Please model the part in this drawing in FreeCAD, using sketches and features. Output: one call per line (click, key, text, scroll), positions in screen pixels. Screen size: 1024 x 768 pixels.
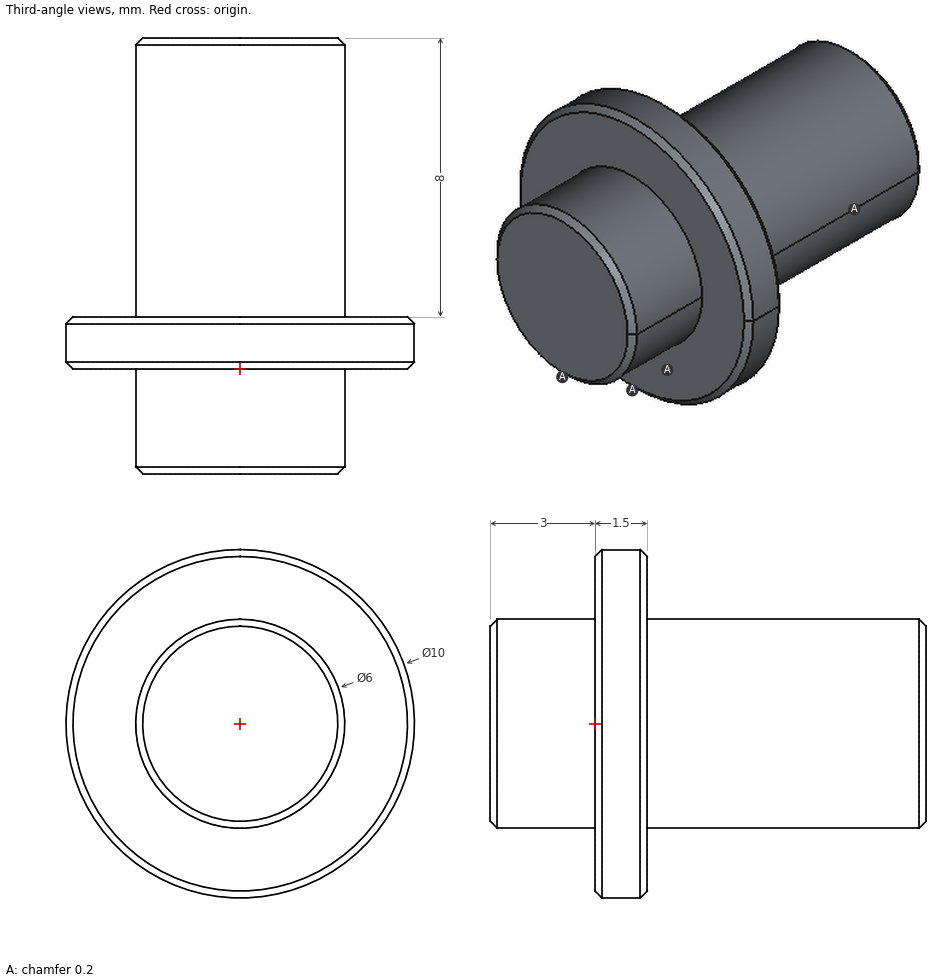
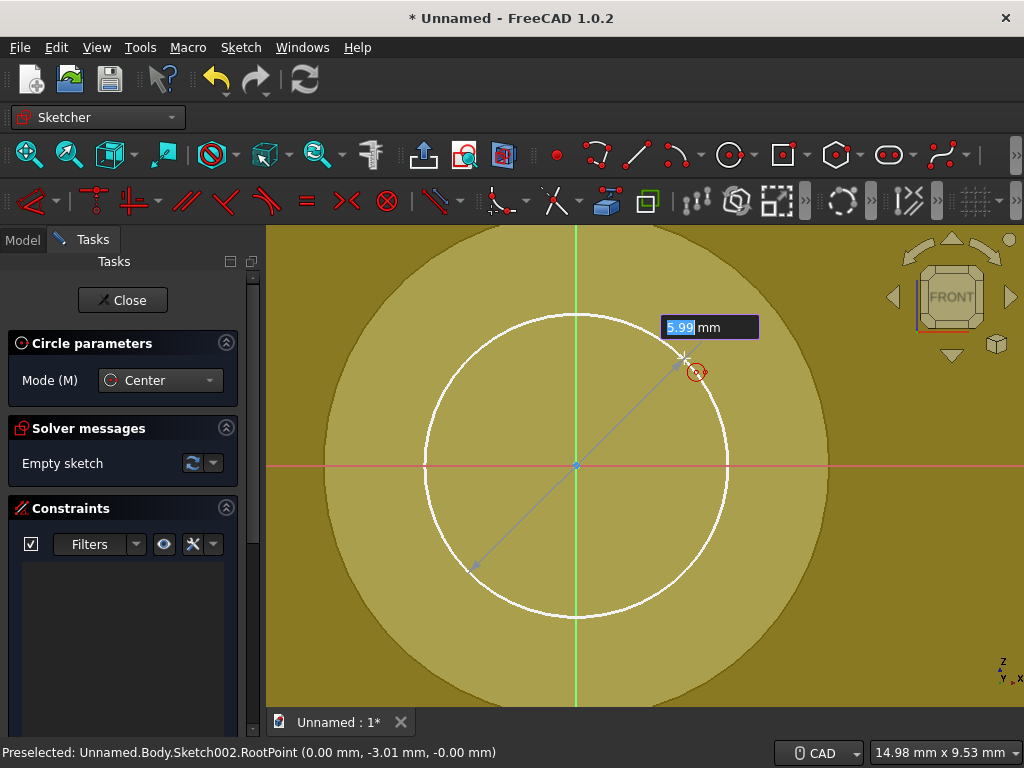
text(6)
key(Return)
key(Escape)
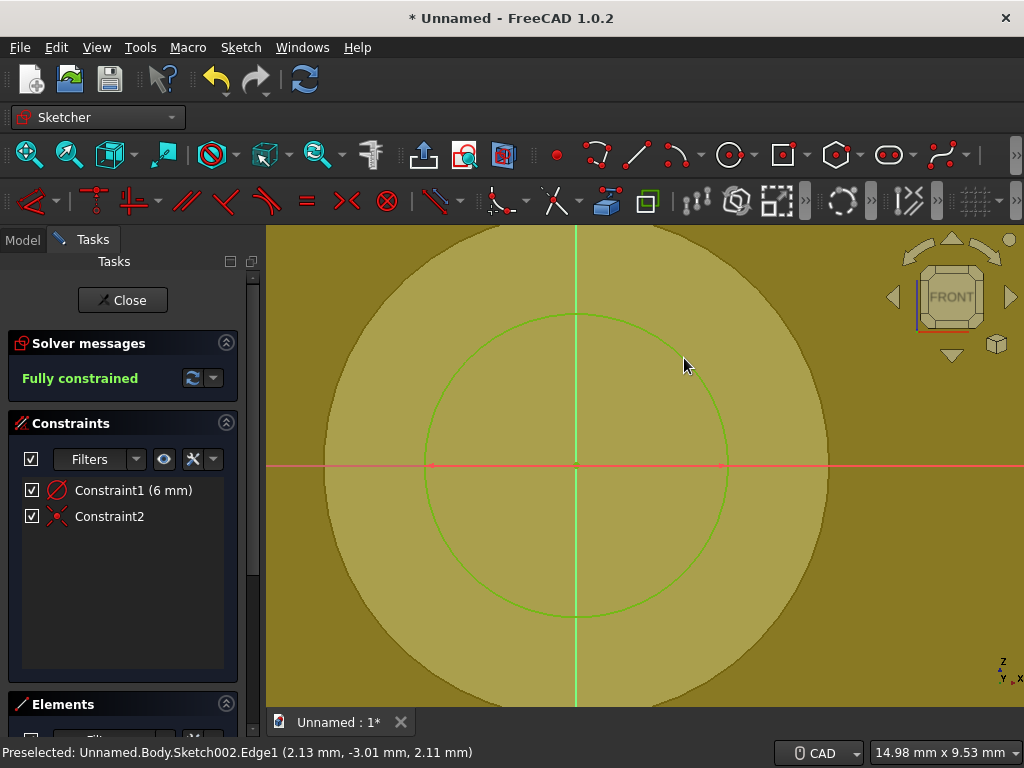
click(123, 300)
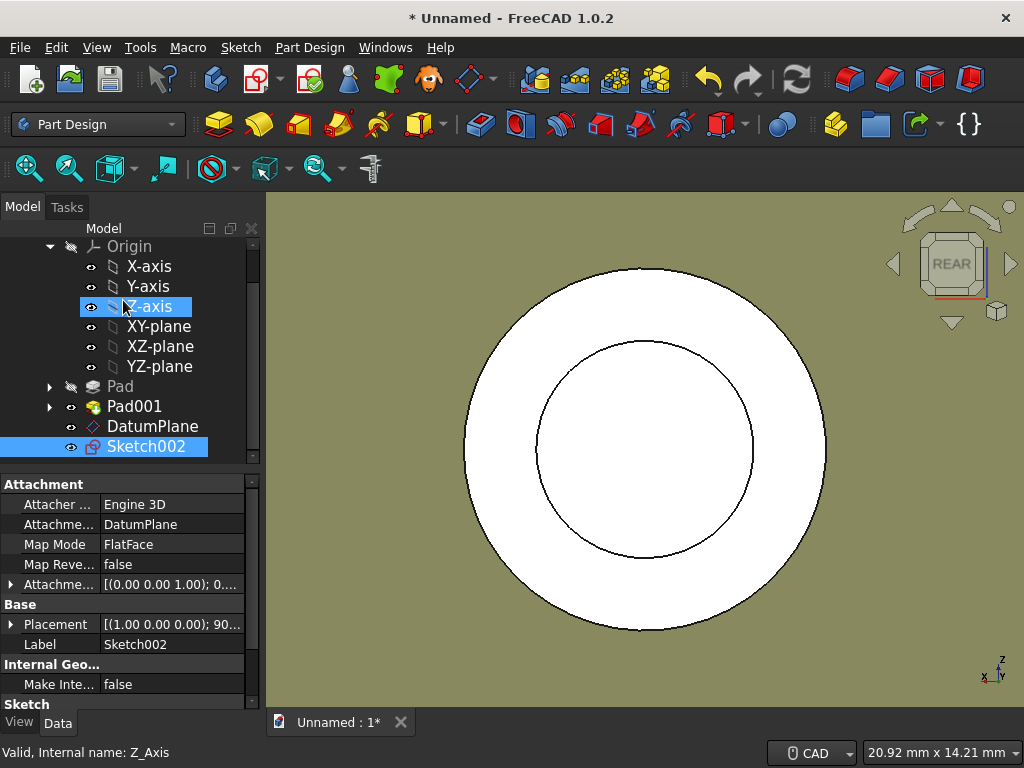
click(220, 124)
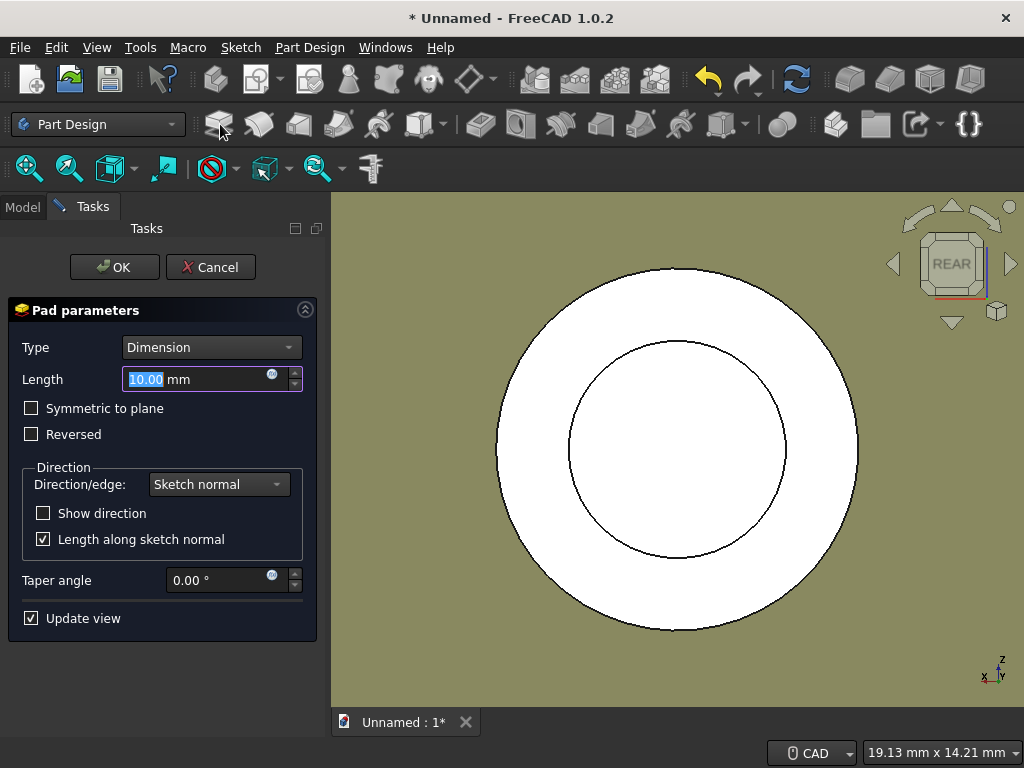
text(3)
key(Tab)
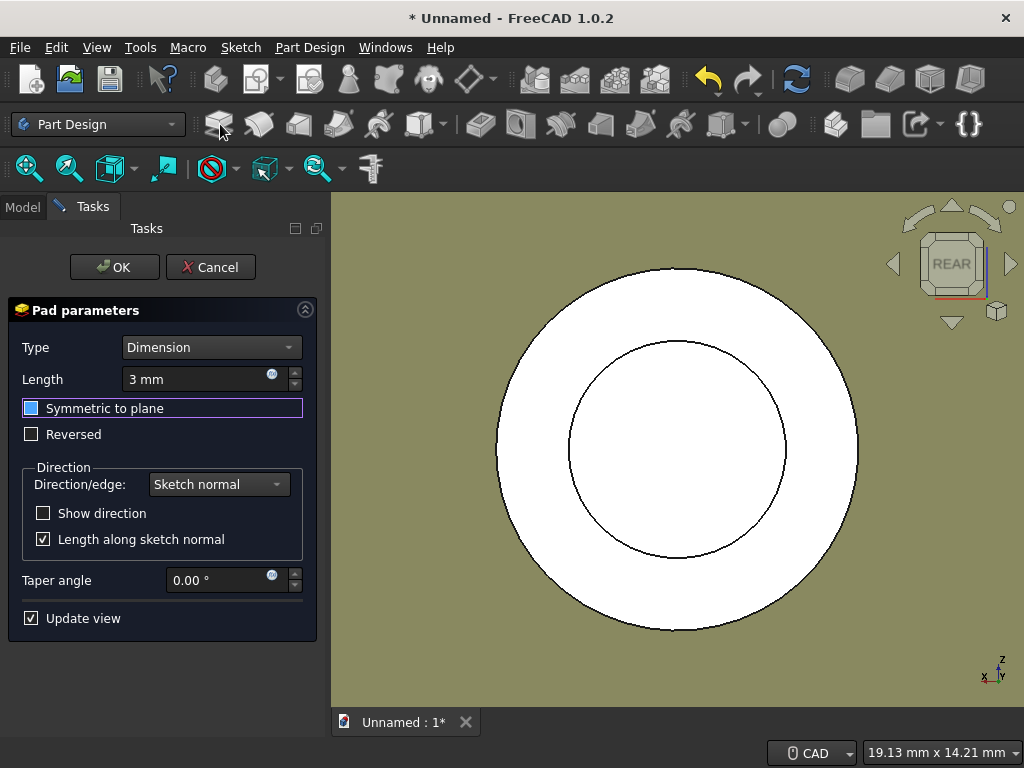
click(30, 434)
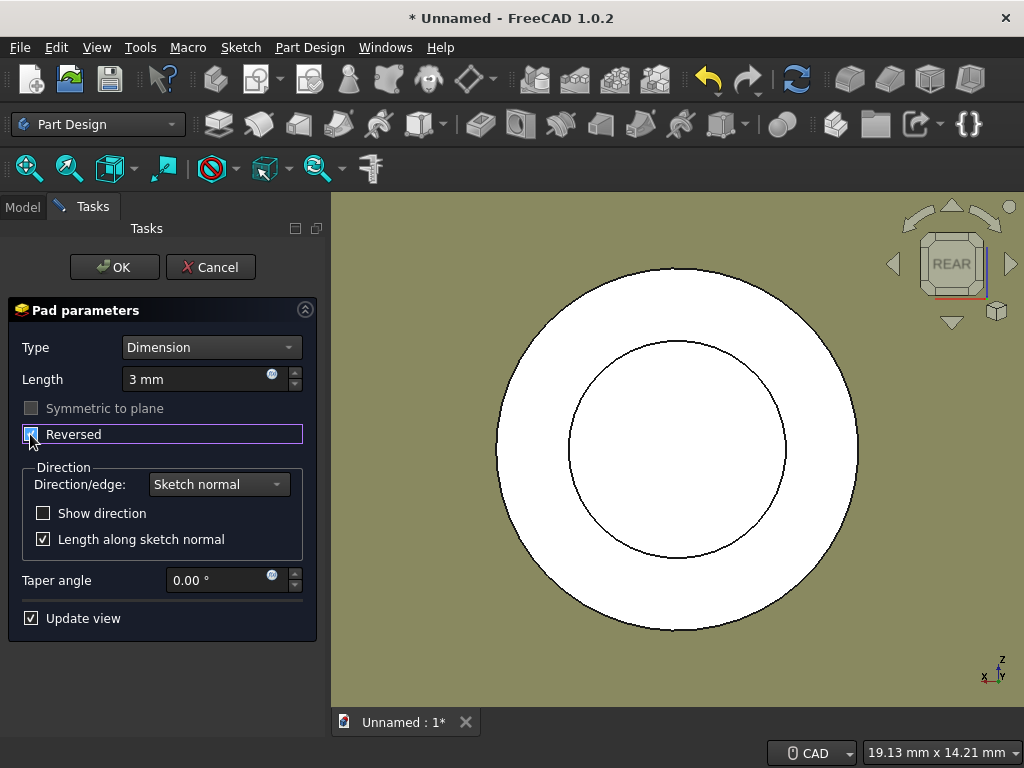
click(115, 267)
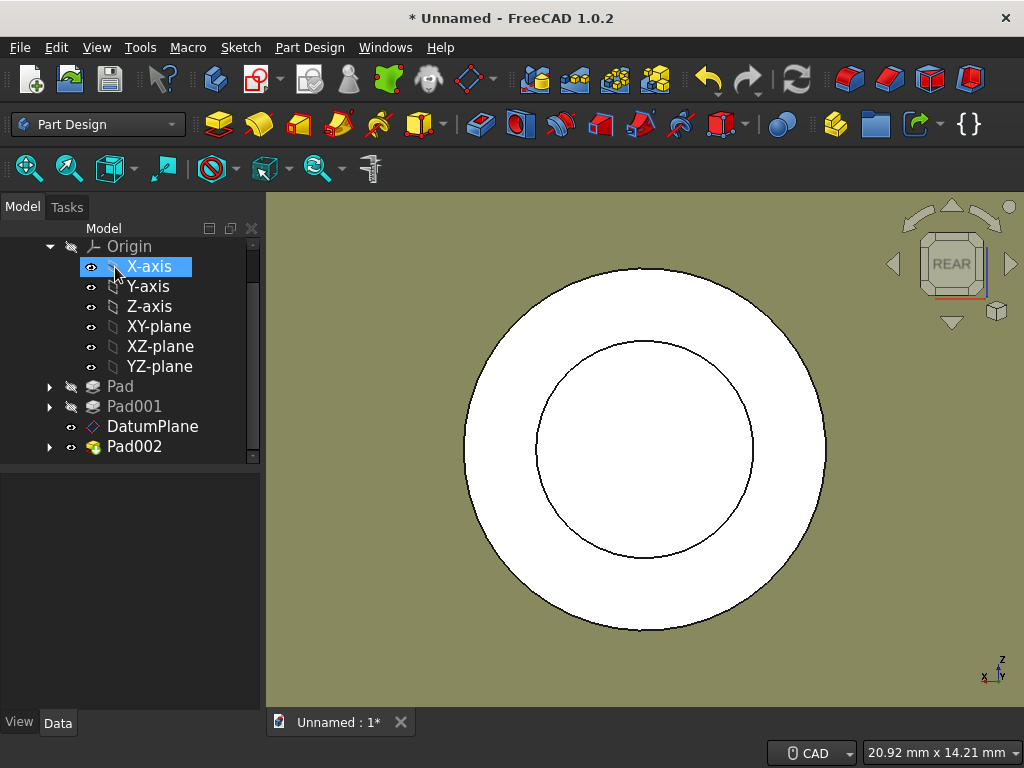
click(116, 427)
key(space)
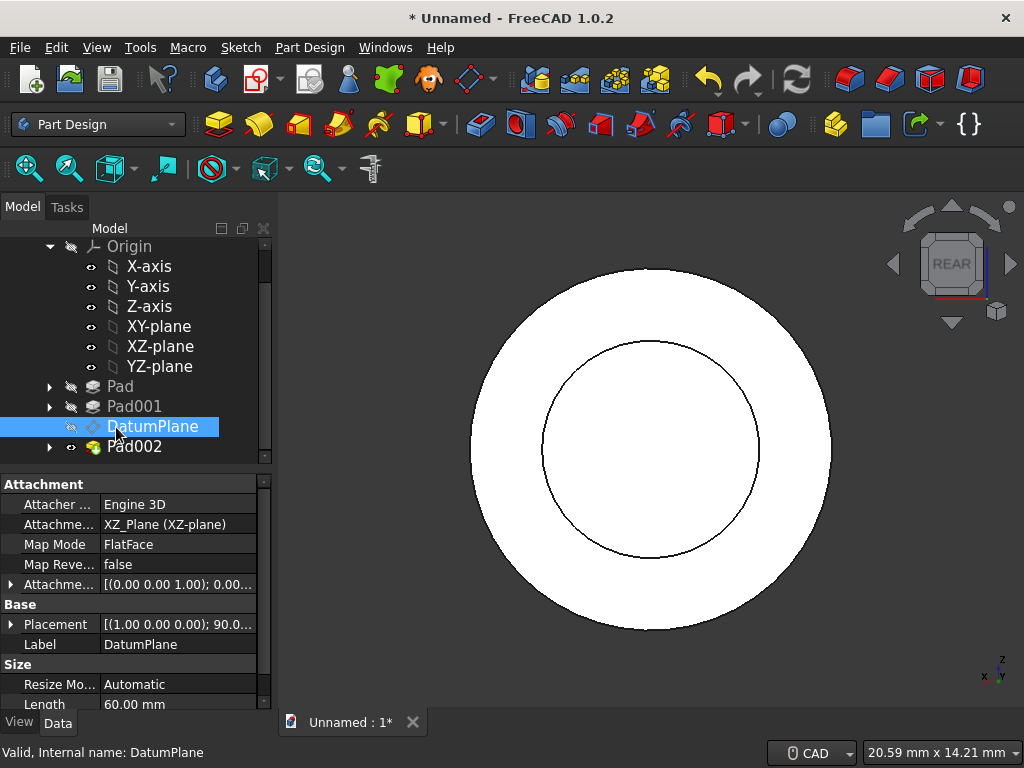
click(832, 448)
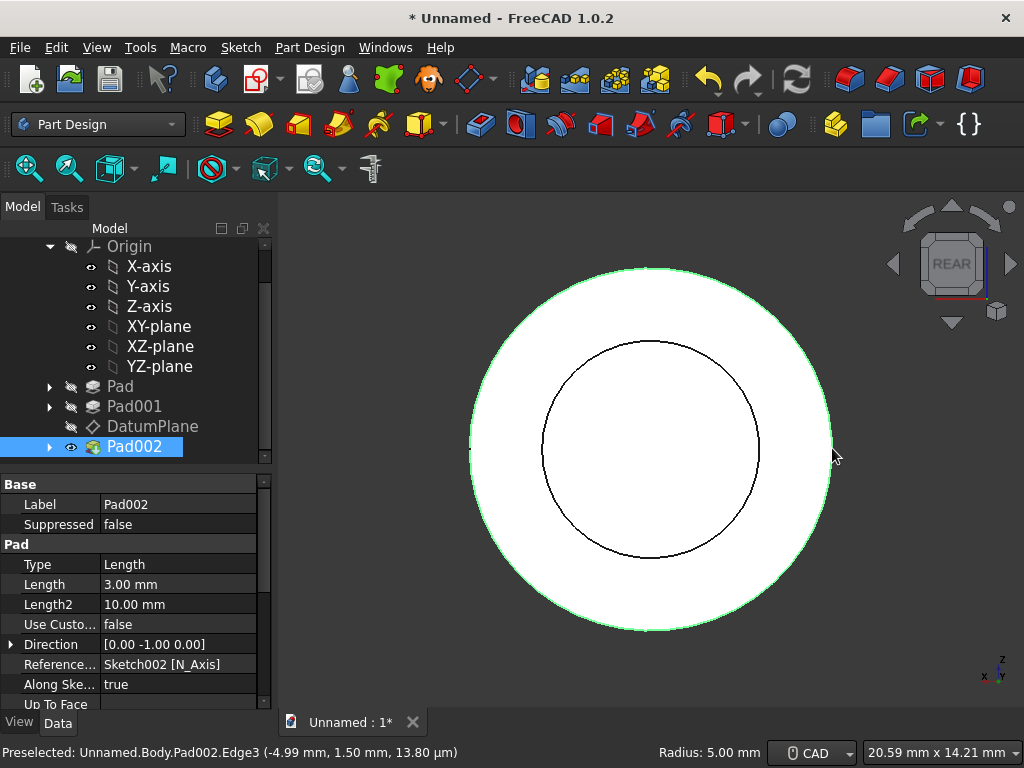
click(759, 448, ctrl)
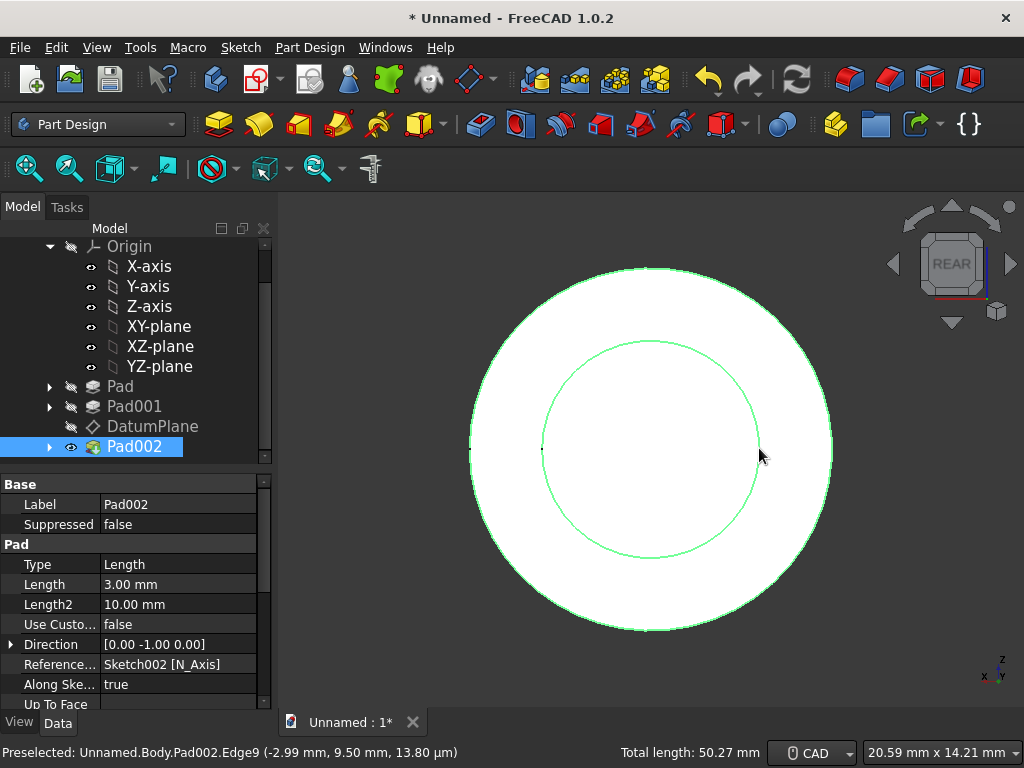
key(0)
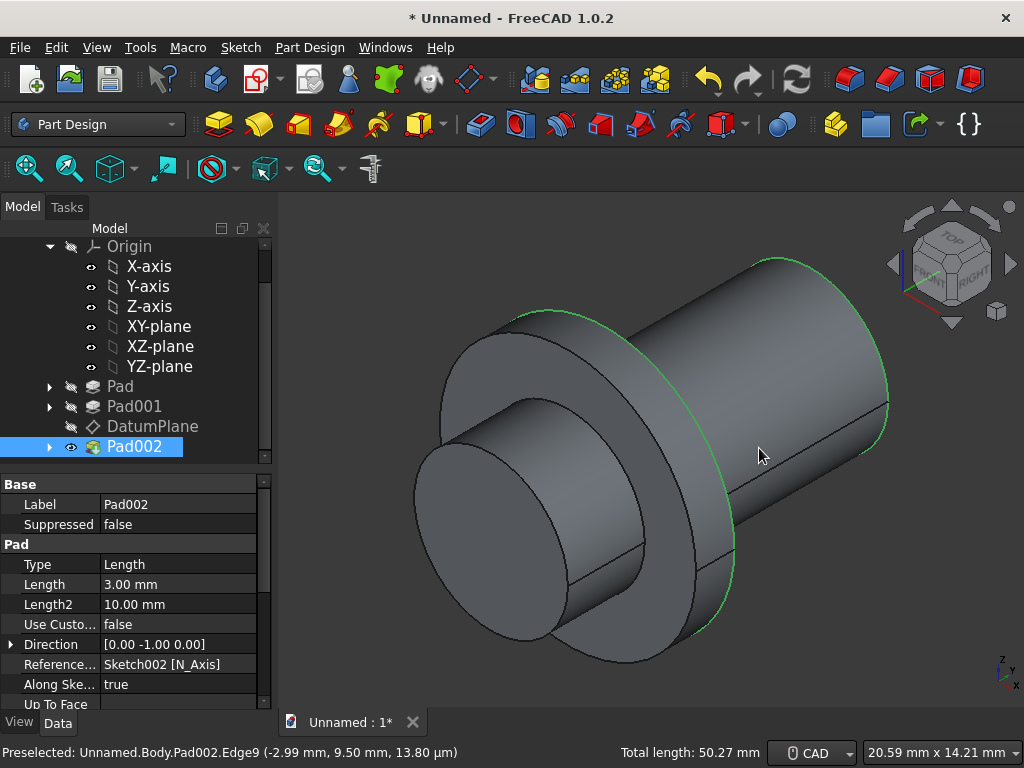
key(v)
key(f)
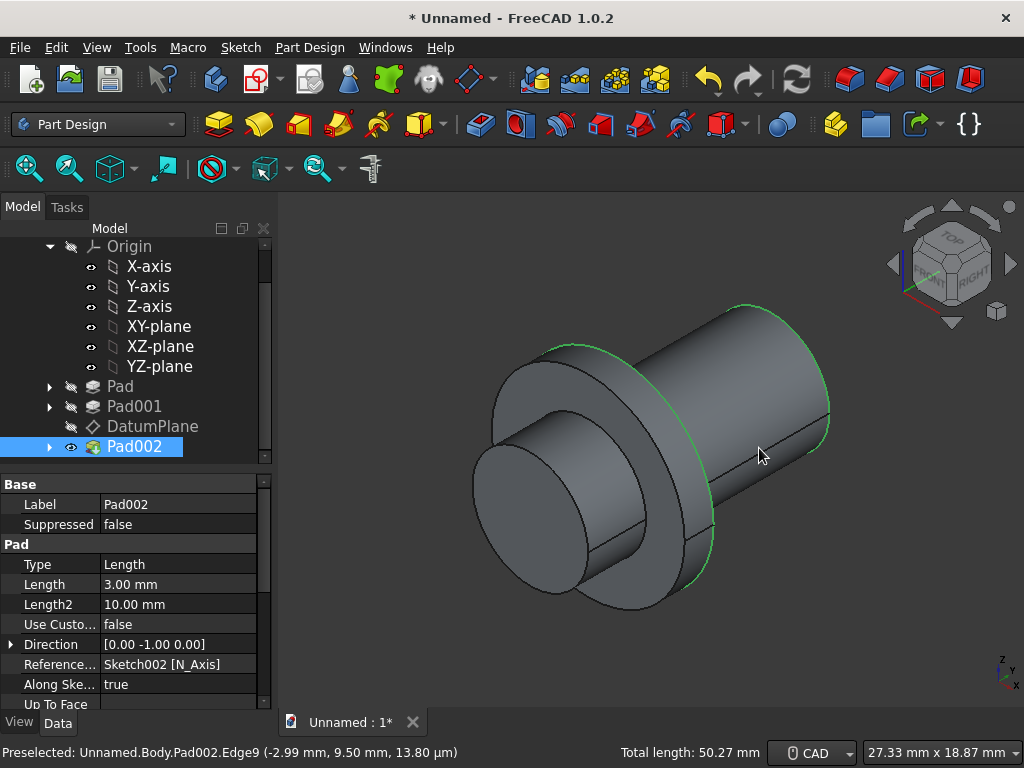
click(512, 444, ctrl)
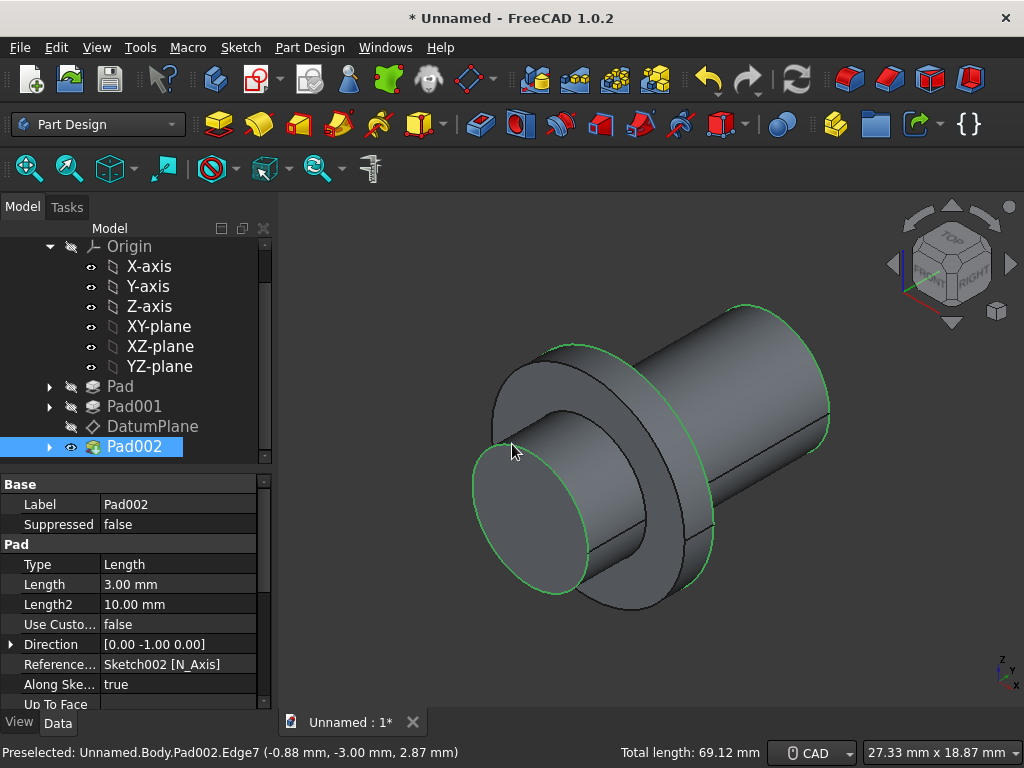
click(558, 361, ctrl)